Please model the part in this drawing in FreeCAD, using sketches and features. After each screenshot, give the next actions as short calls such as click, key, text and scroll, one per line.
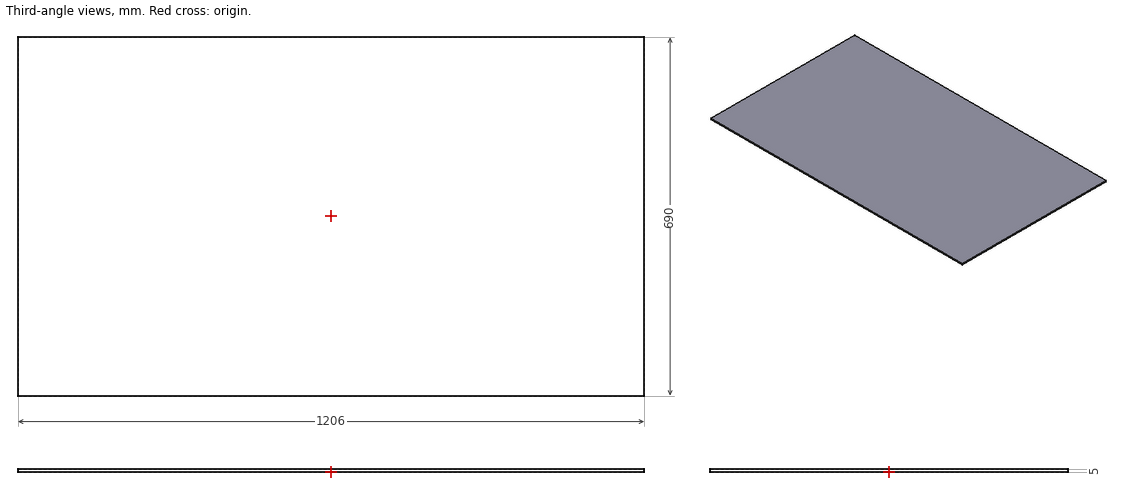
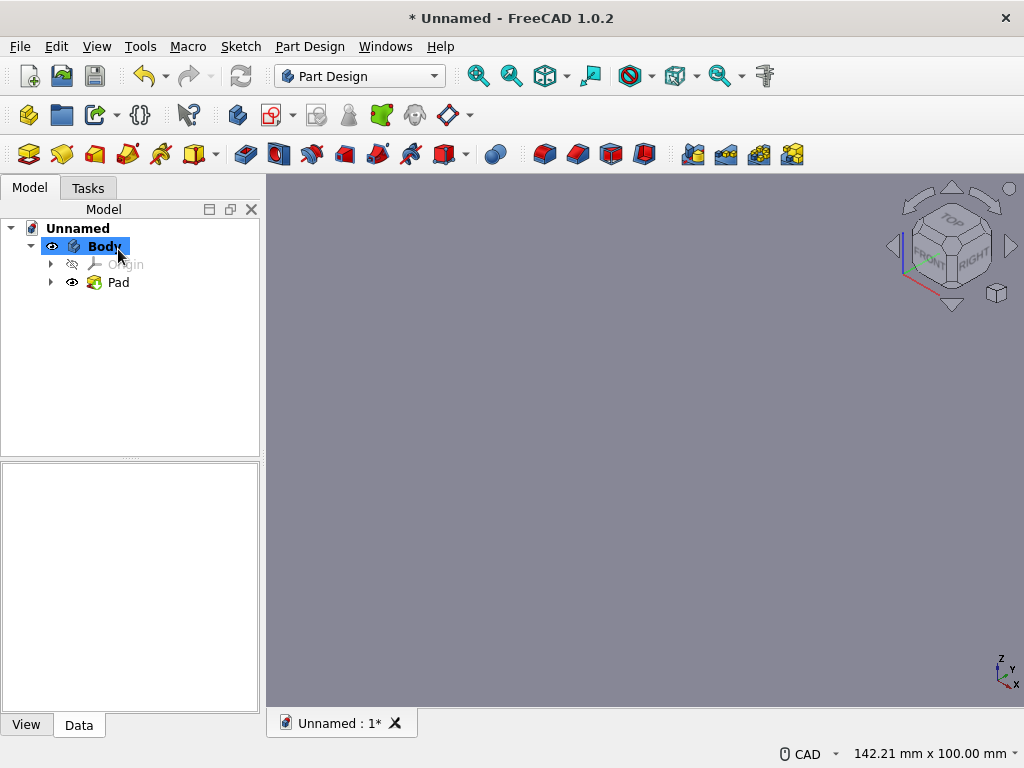
key(v)
key(f)